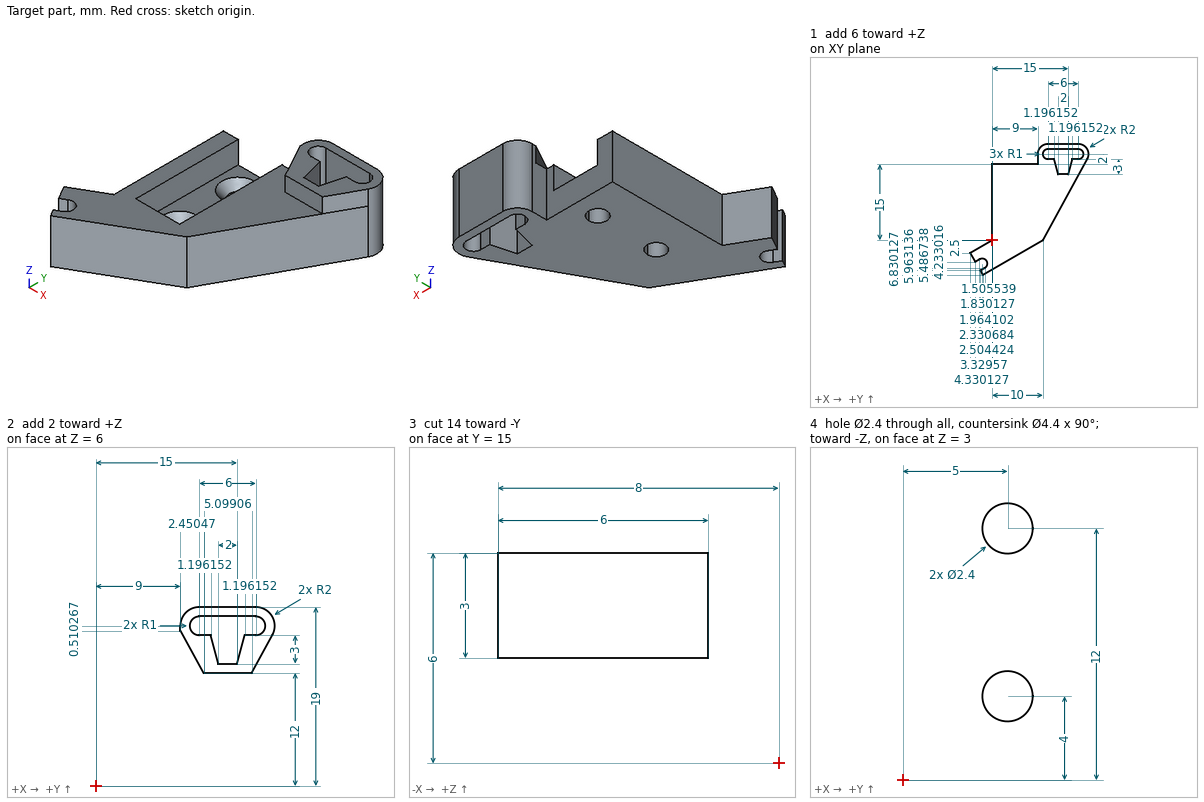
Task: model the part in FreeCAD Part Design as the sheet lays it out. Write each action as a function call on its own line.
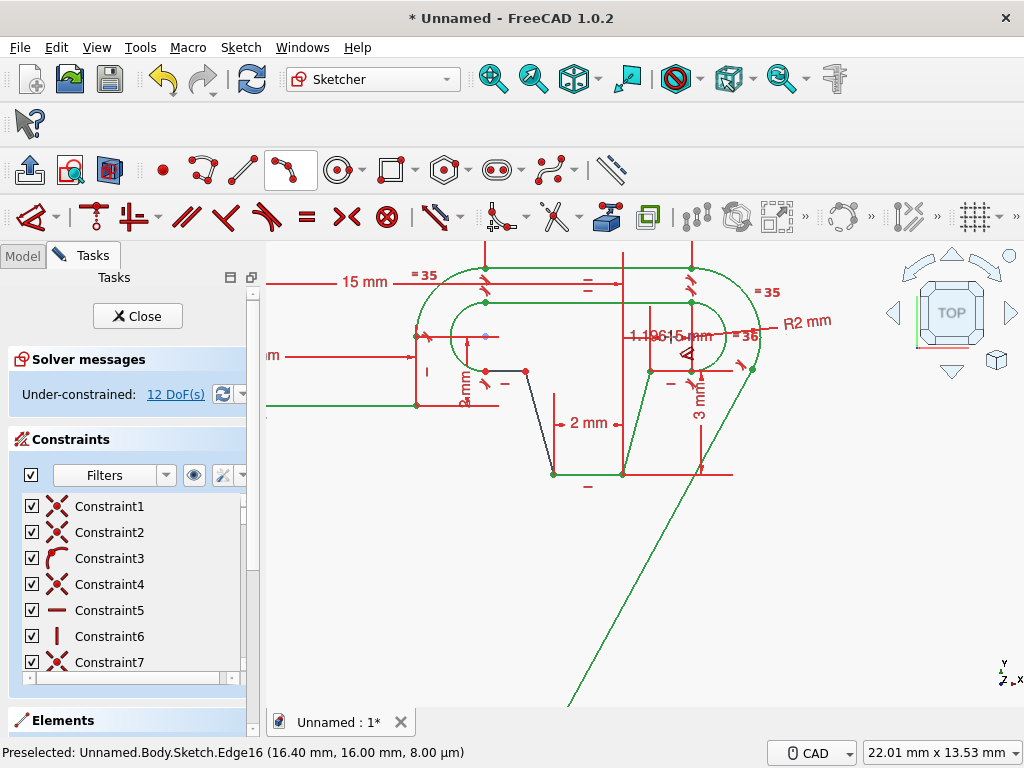
click(513, 371)
click(505, 337)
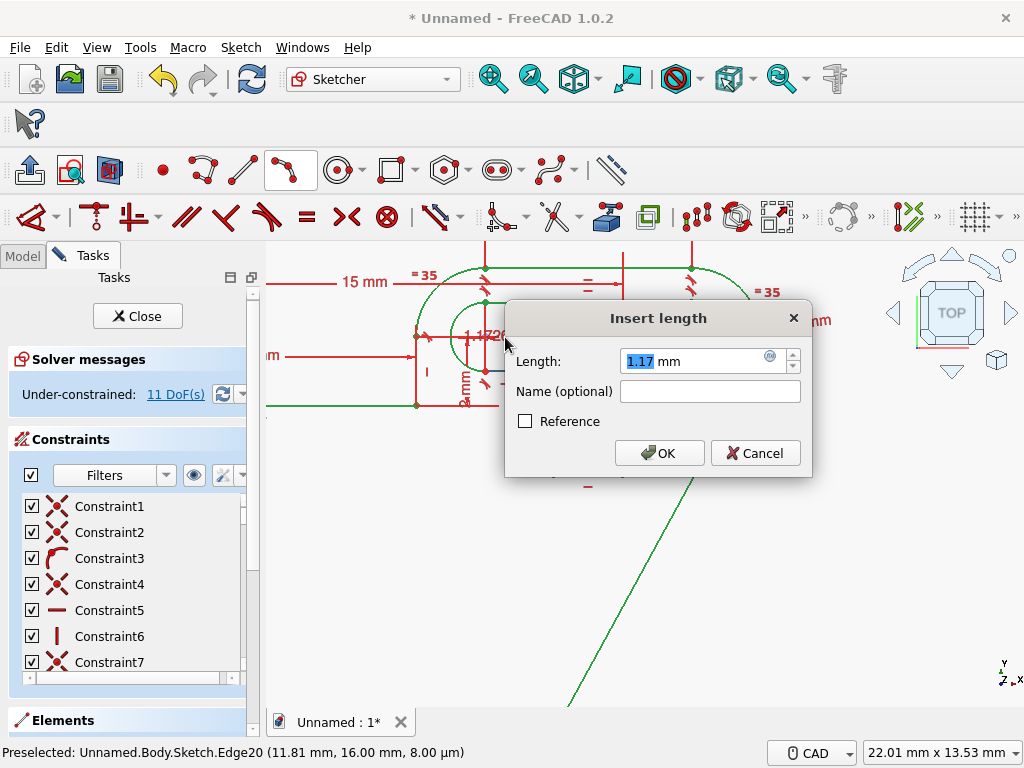
text(1.196152)
key(Return)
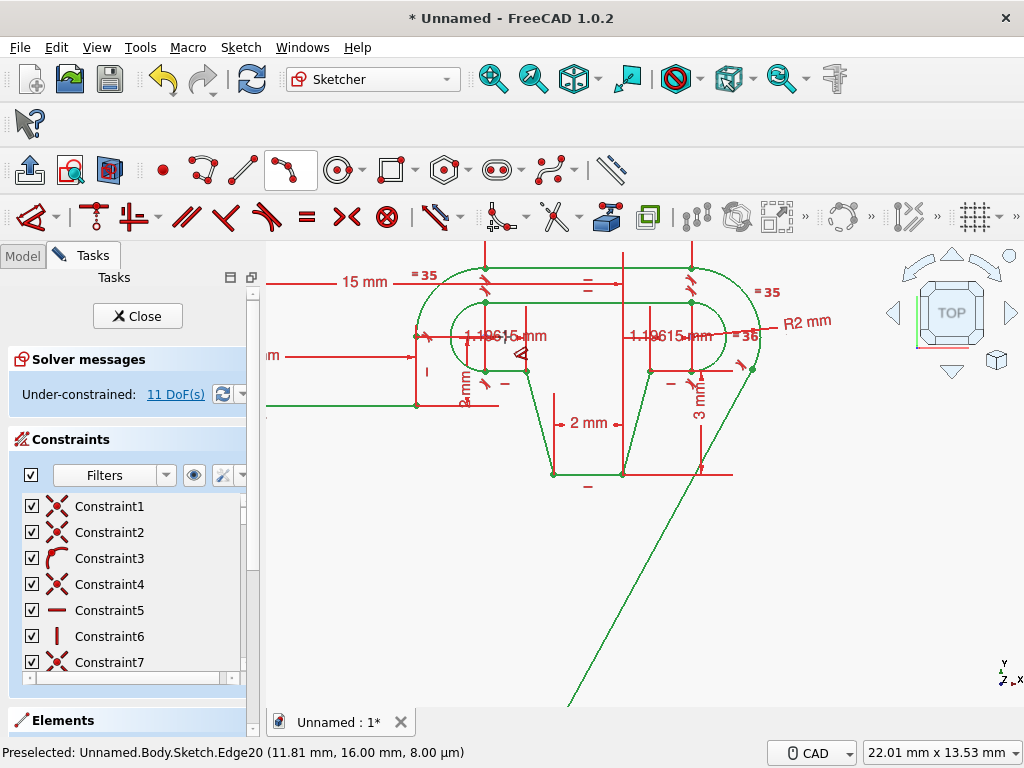
scroll(672, 371, down, 6)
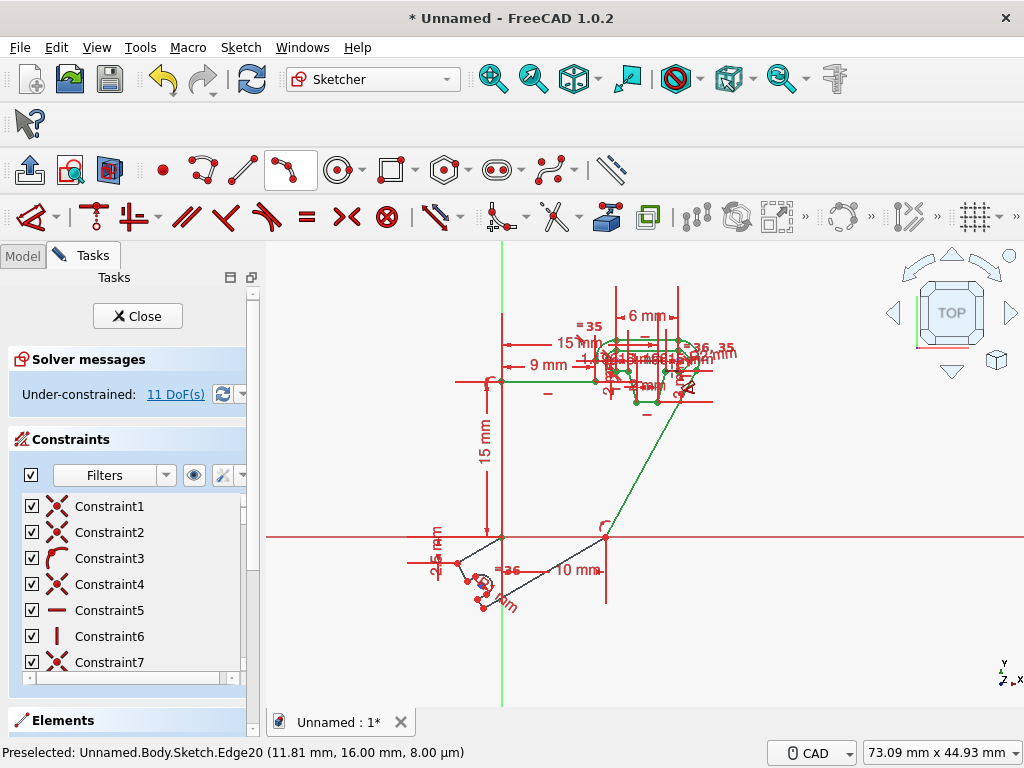
scroll(467, 582, up, 2)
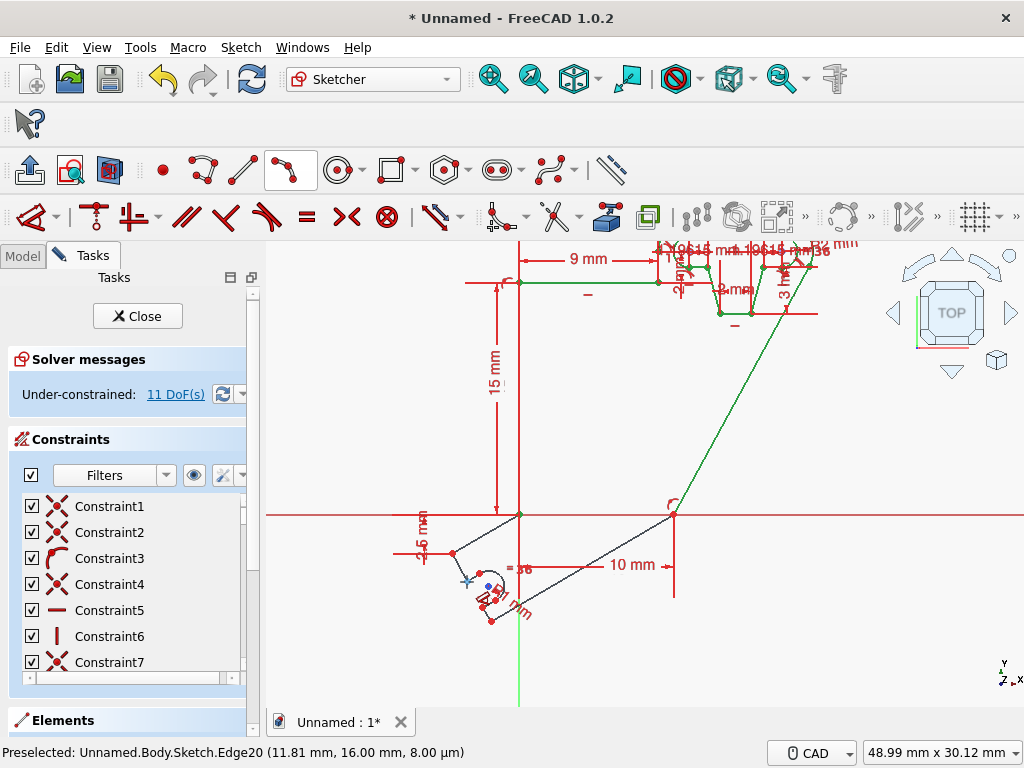
click(467, 581)
click(493, 481)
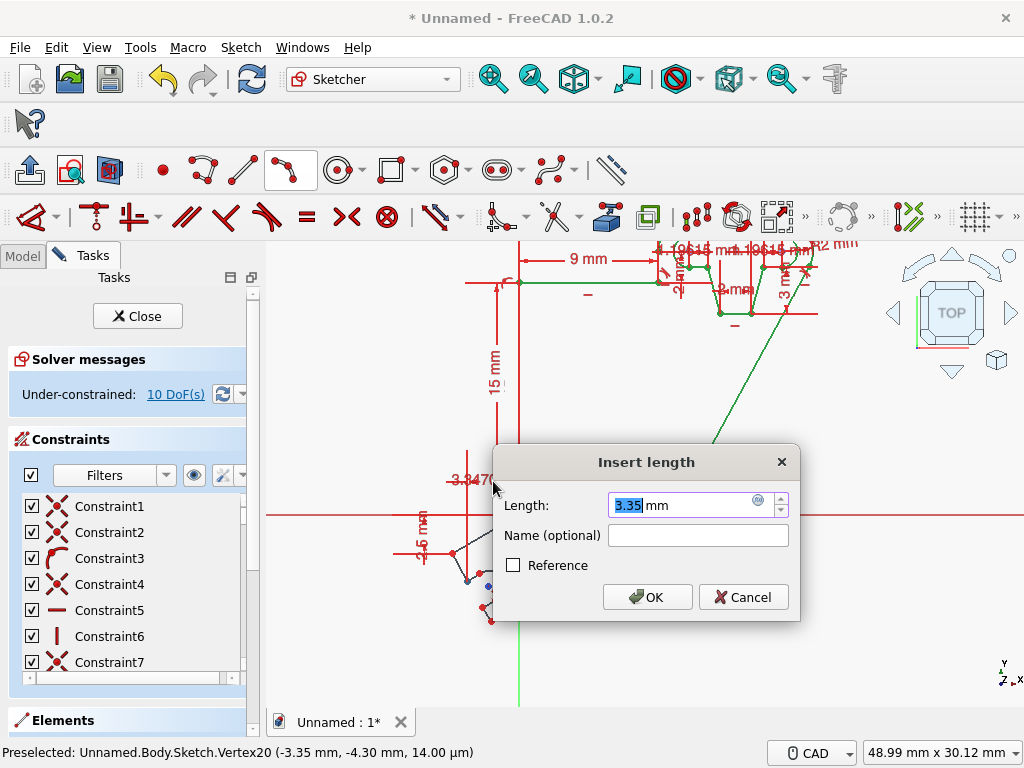
text(3.32957)
key(Return)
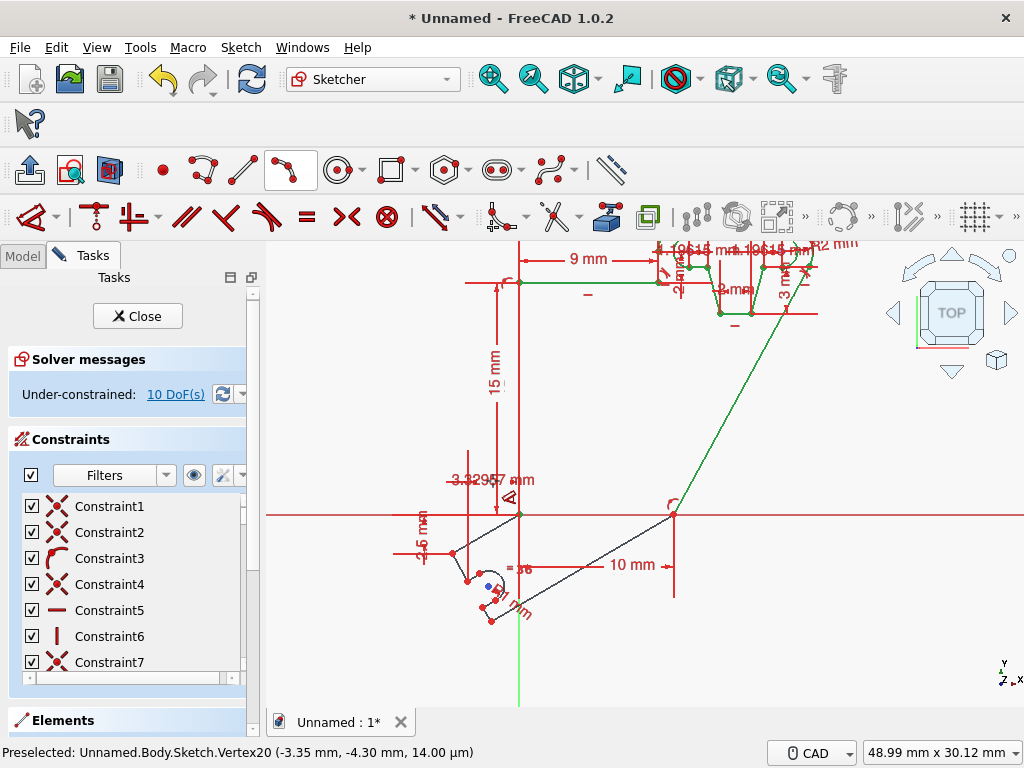
scroll(496, 600, up, 3)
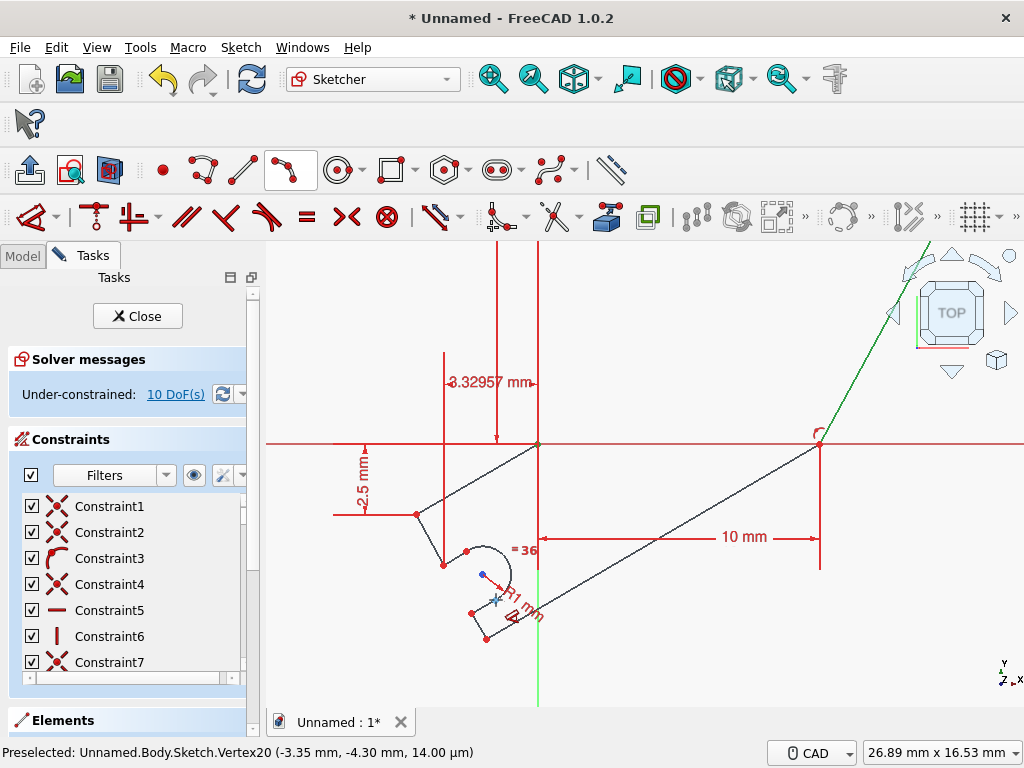
click(495, 600)
click(516, 410)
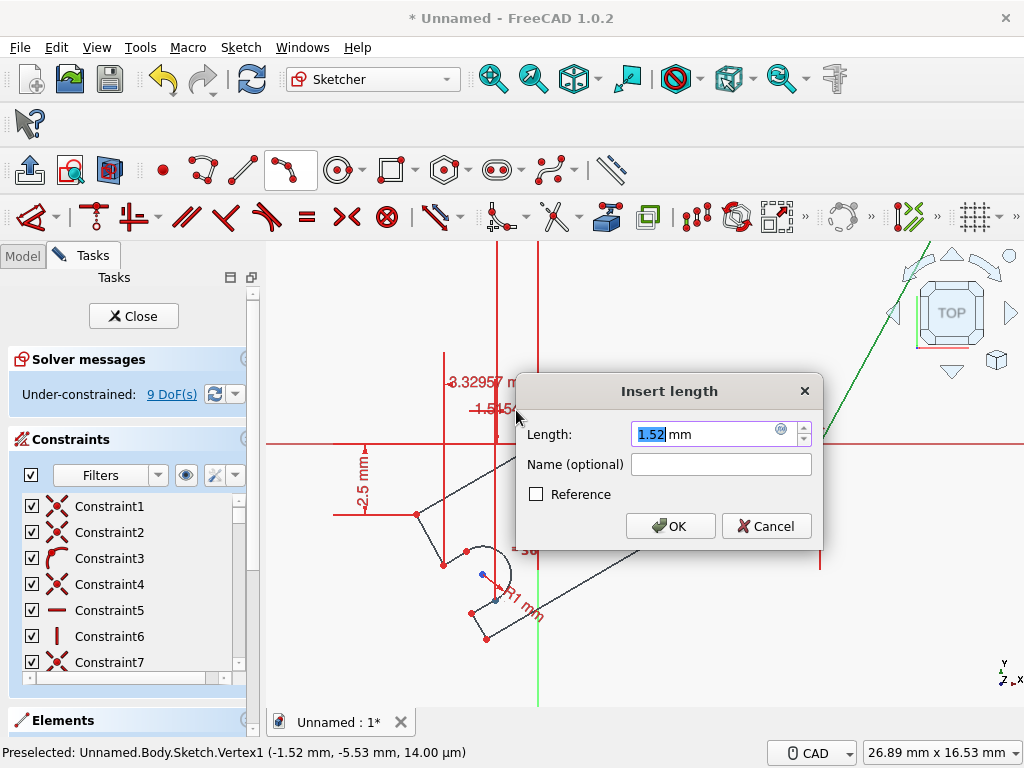
text(1.505539)
key(Return)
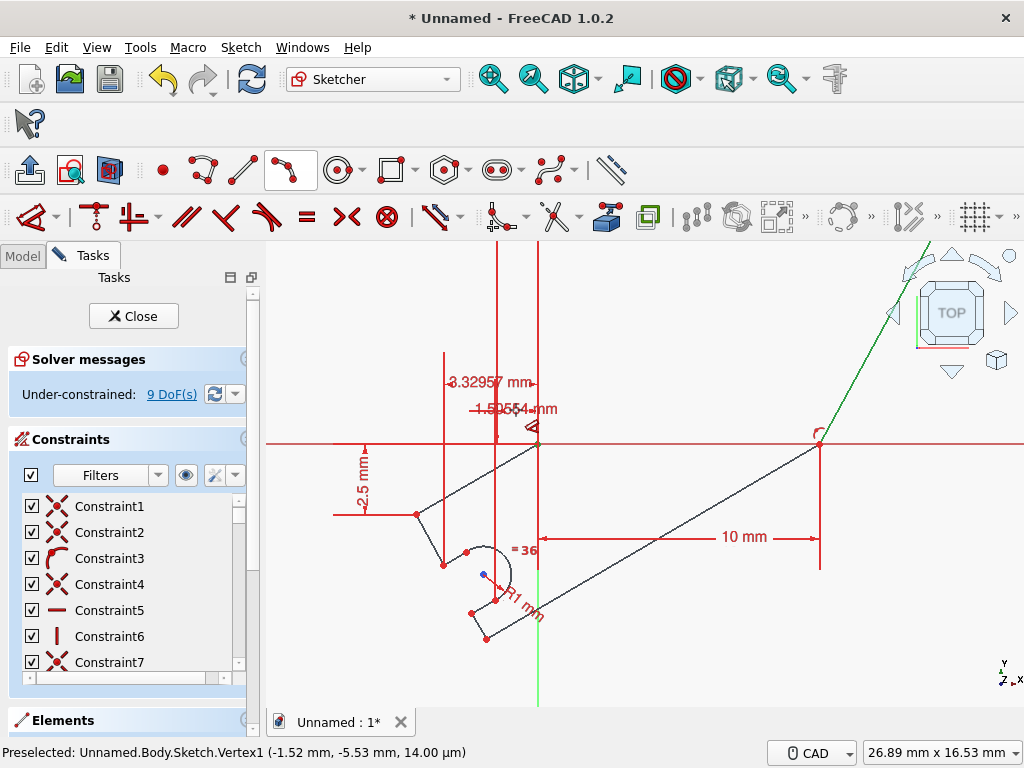
click(495, 600)
click(461, 522)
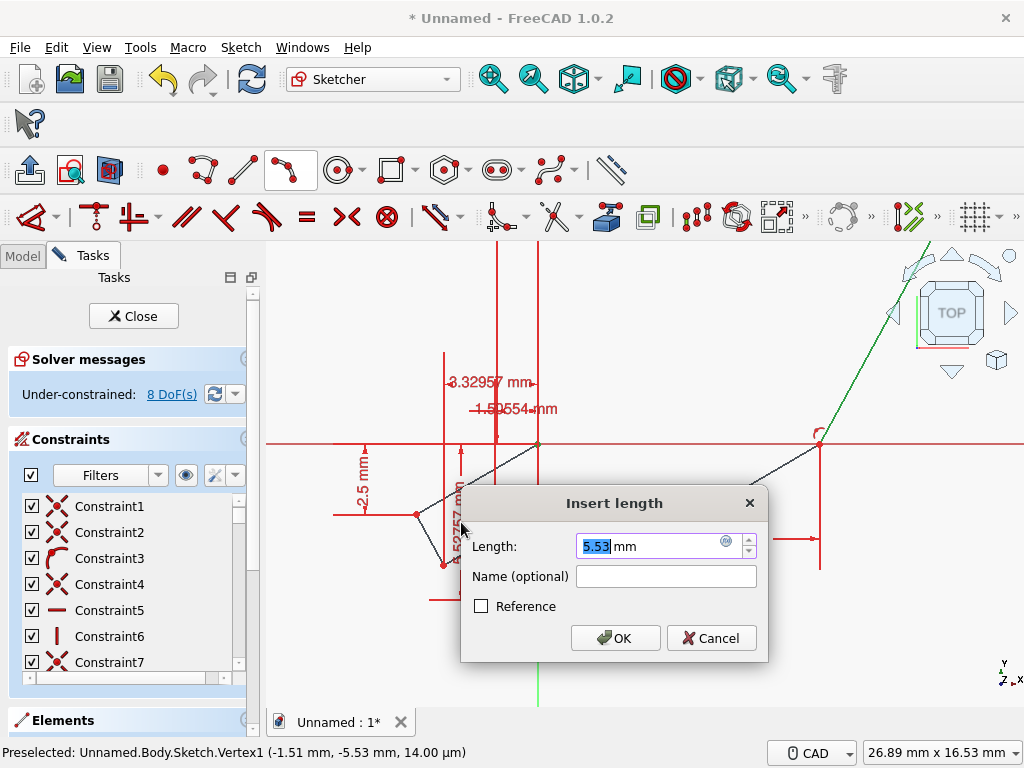
text(5.486738)
key(Return)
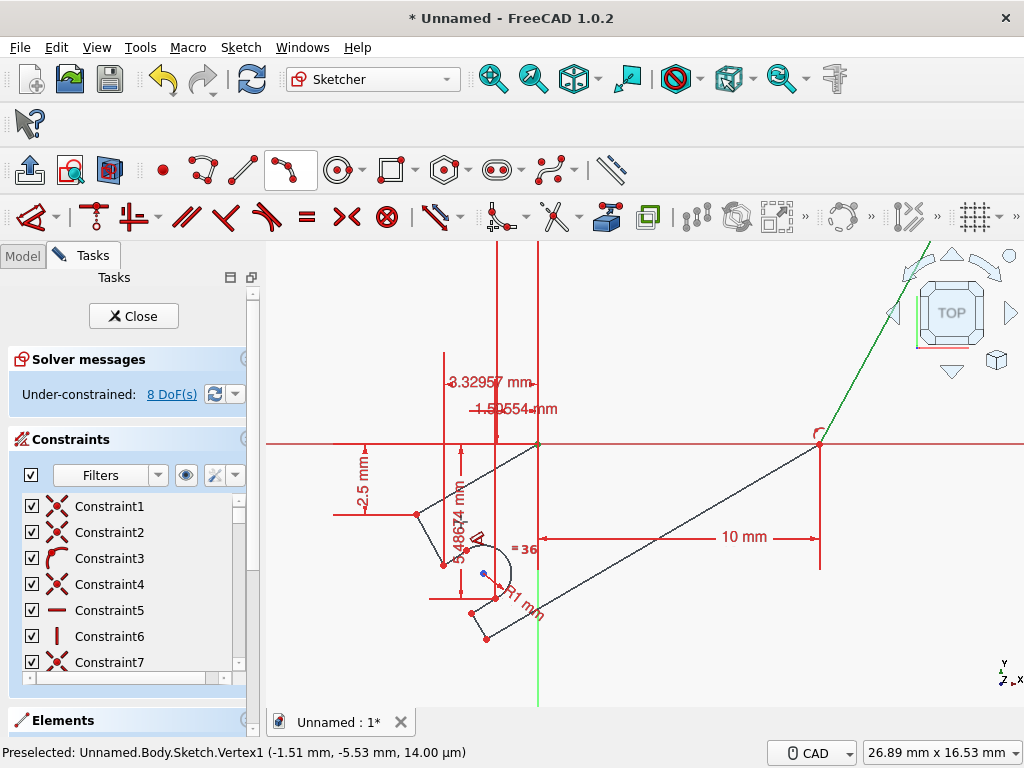
click(472, 614)
click(505, 648)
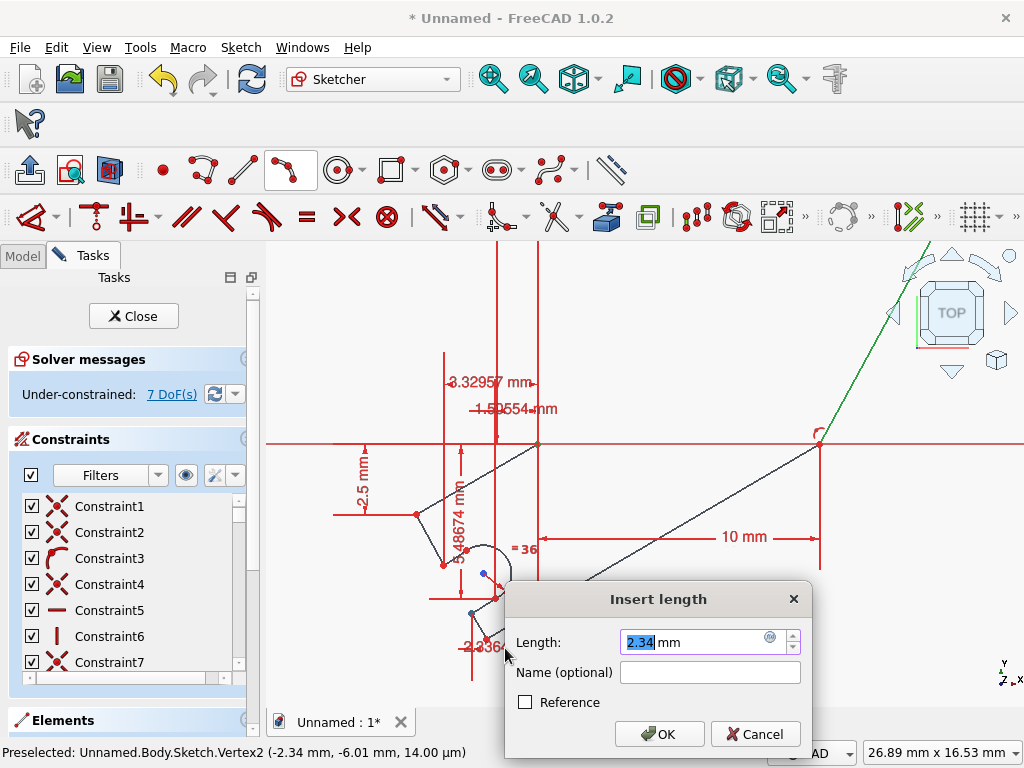
text(2.330684)
key(Return)